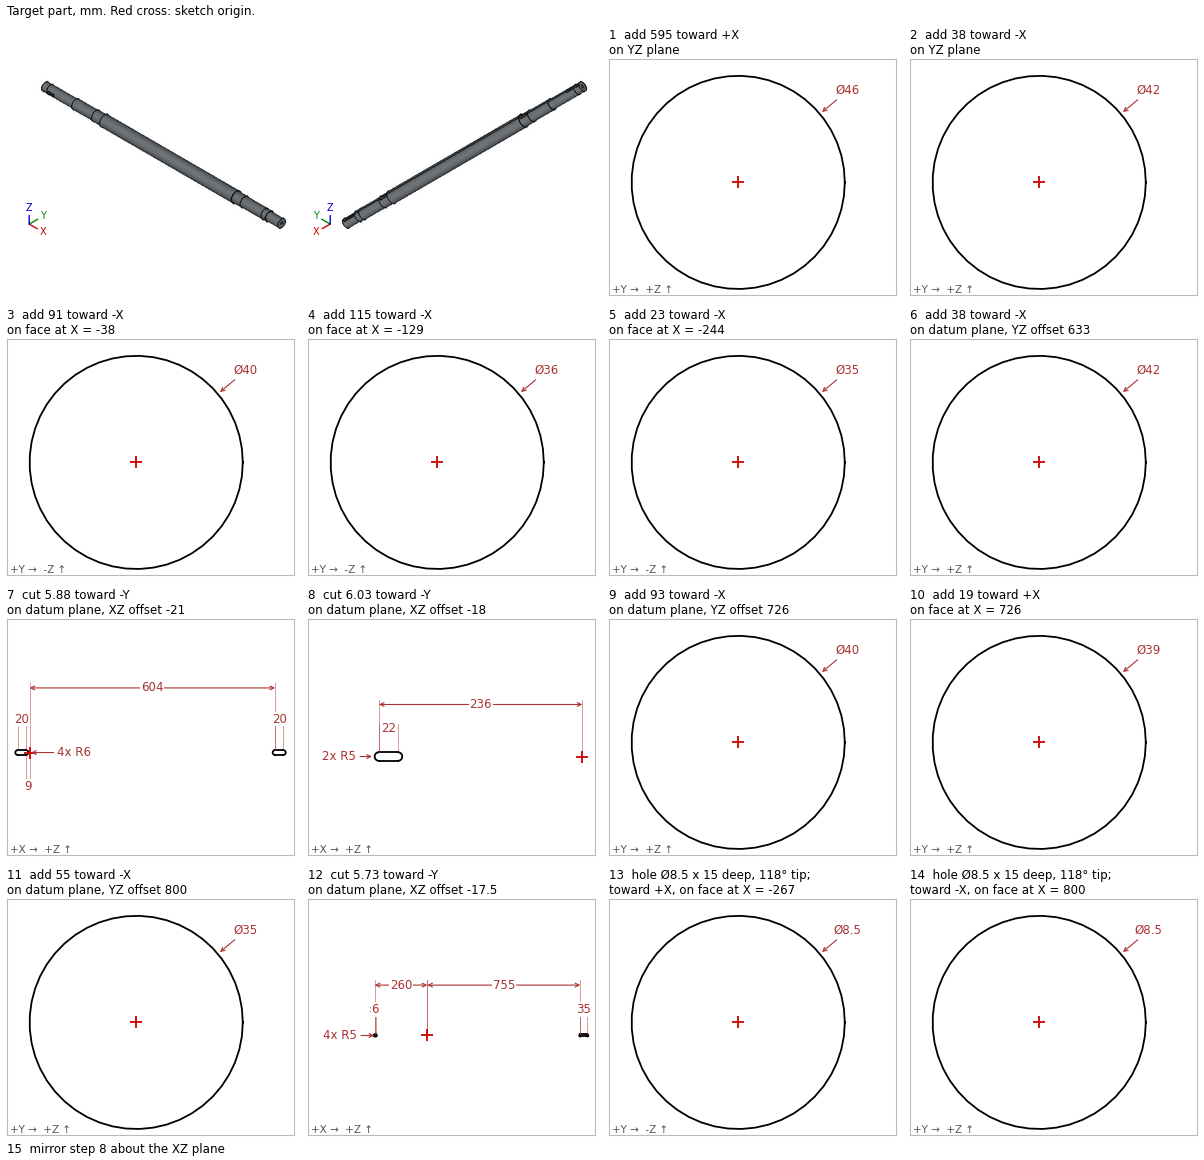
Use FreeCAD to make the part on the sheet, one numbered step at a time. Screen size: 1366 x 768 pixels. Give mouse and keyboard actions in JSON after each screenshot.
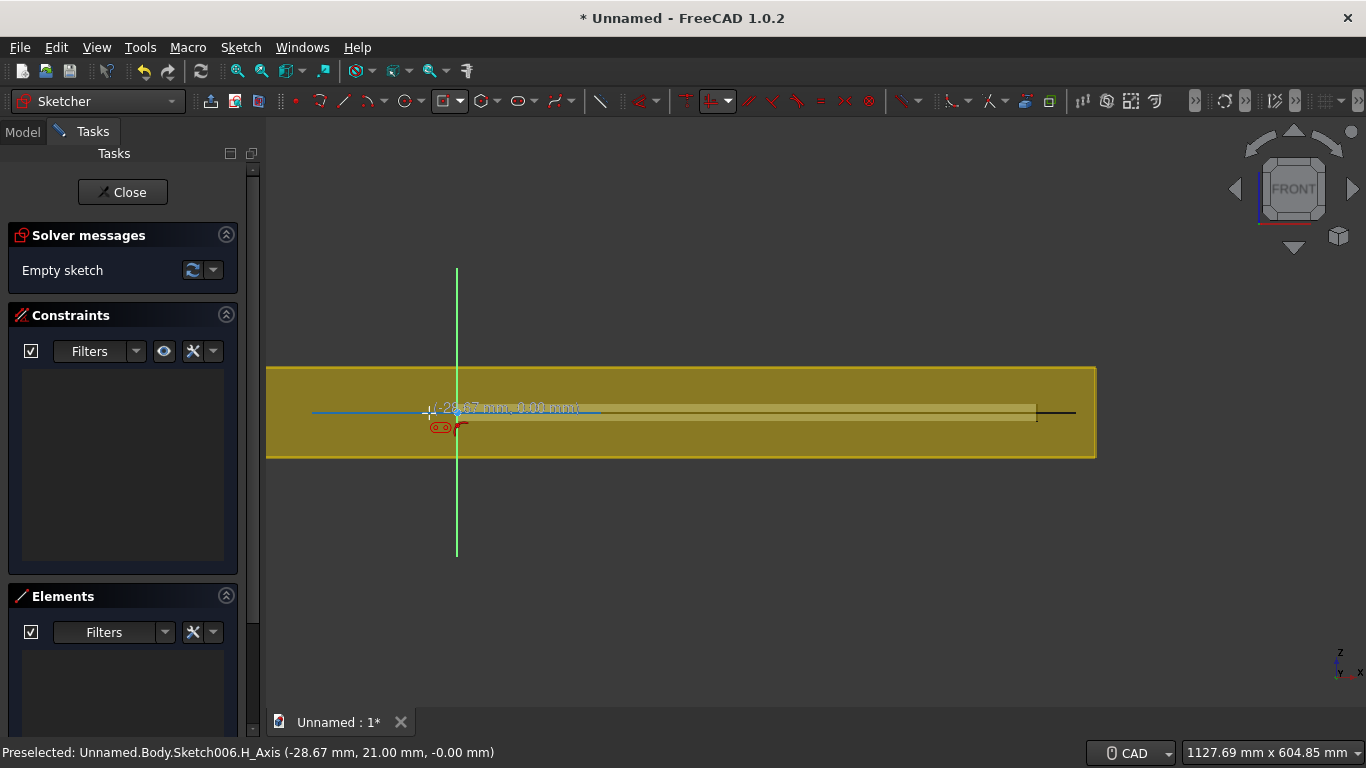
{"action": "left_click", "coordinate": [429, 413]}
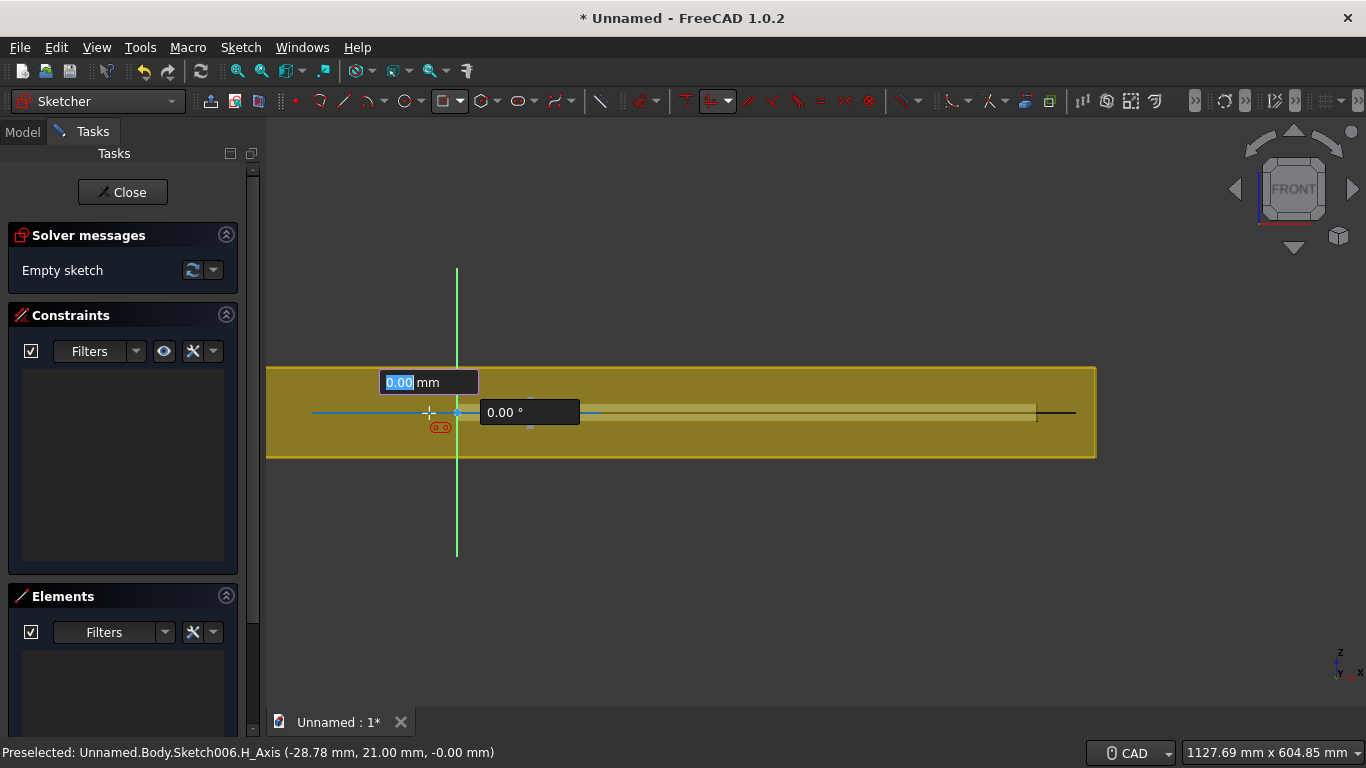
{"action": "scroll", "coordinate": [448, 413], "scroll_direction": "up", "scroll_amount": 3}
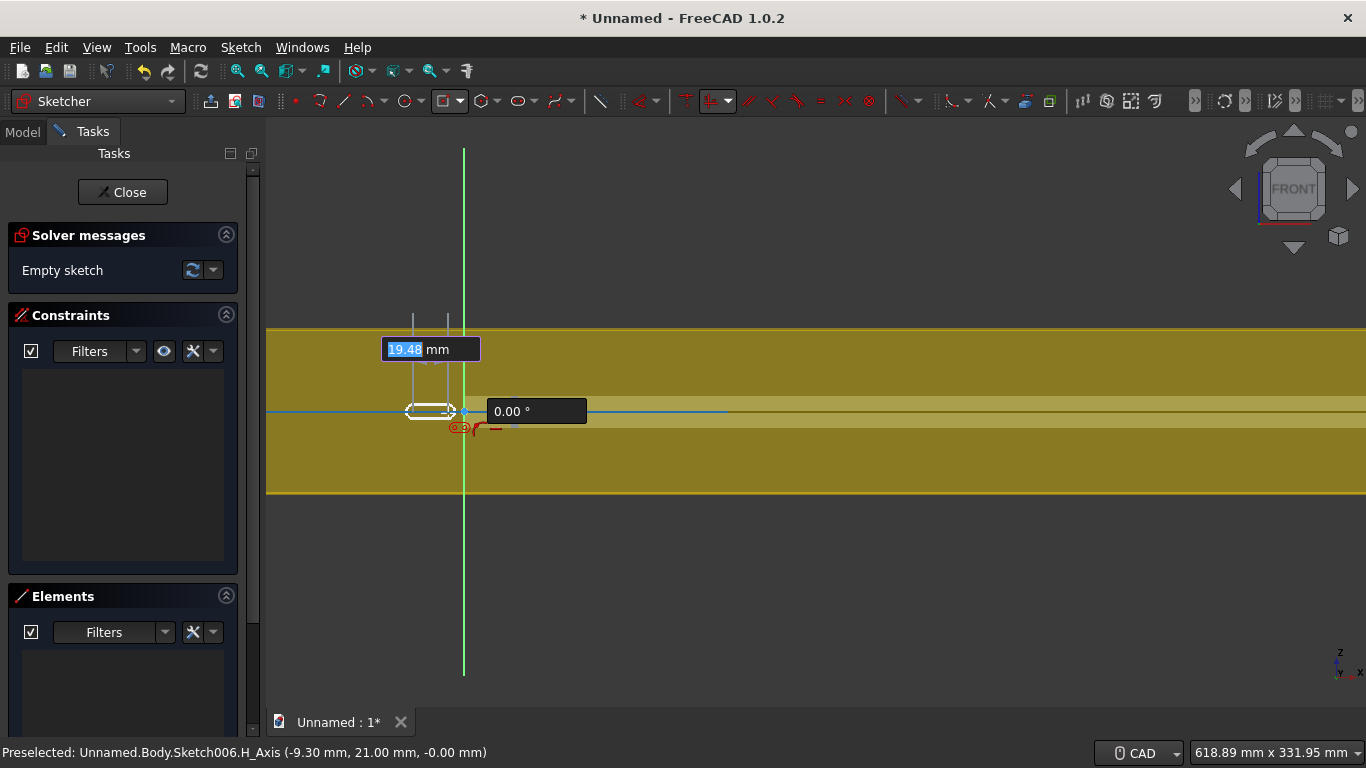
{"action": "left_click", "coordinate": [448, 403]}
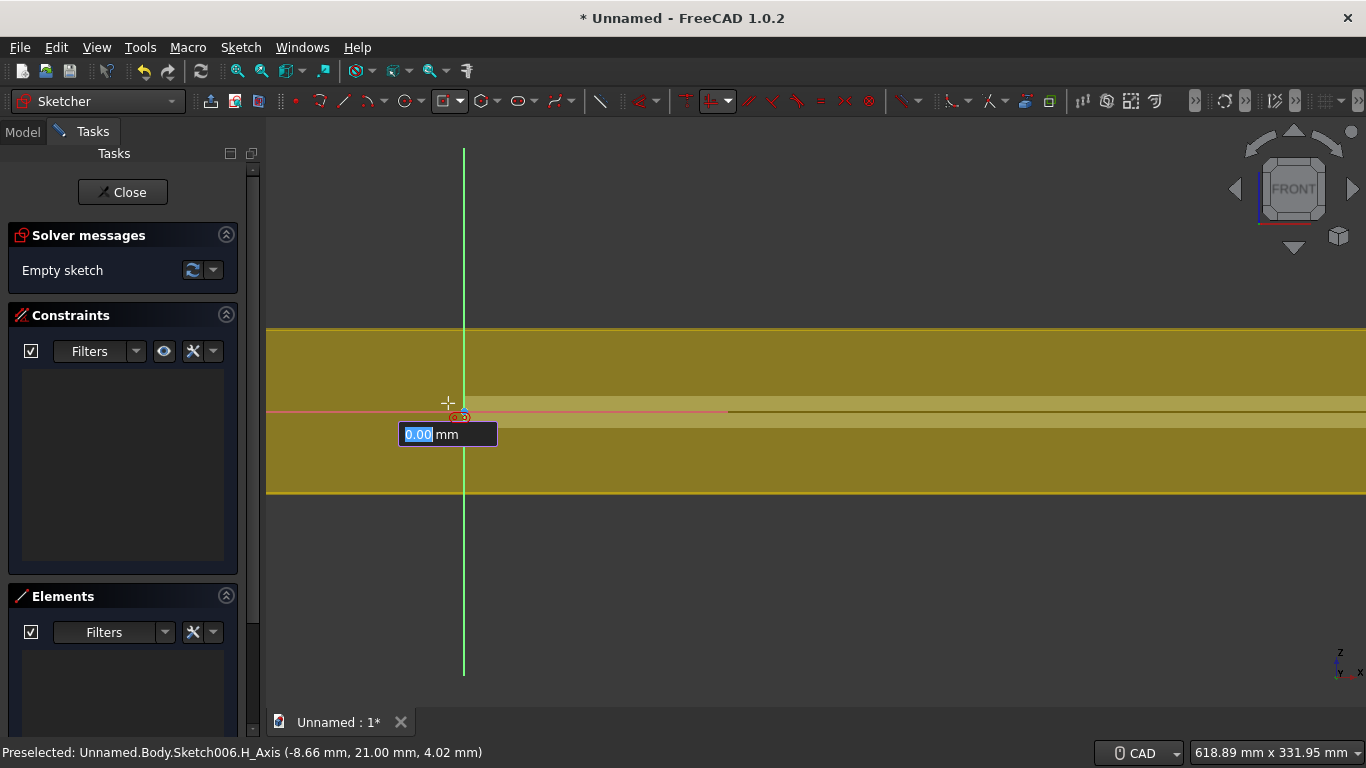
{"action": "scroll", "coordinate": [431, 401], "scroll_direction": "up", "scroll_amount": 2}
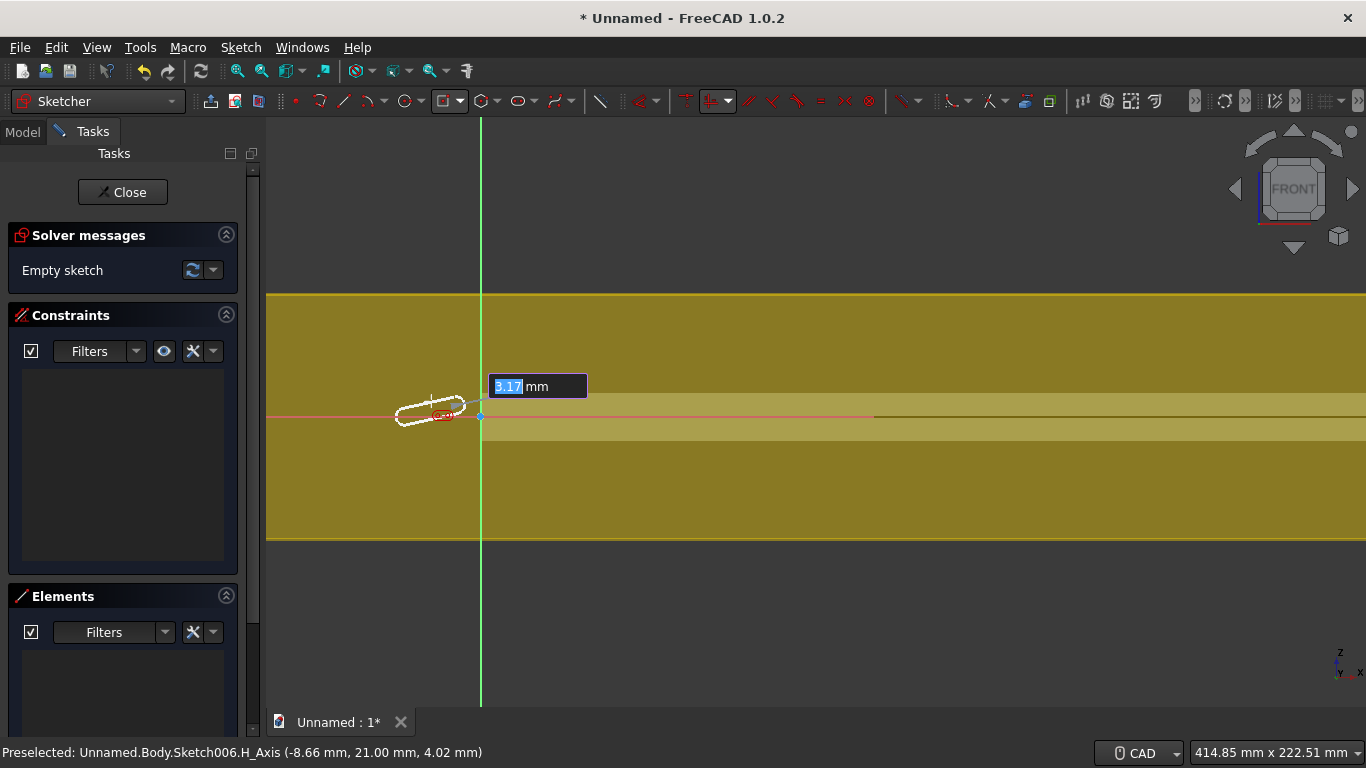
{"action": "left_click", "coordinate": [430, 401]}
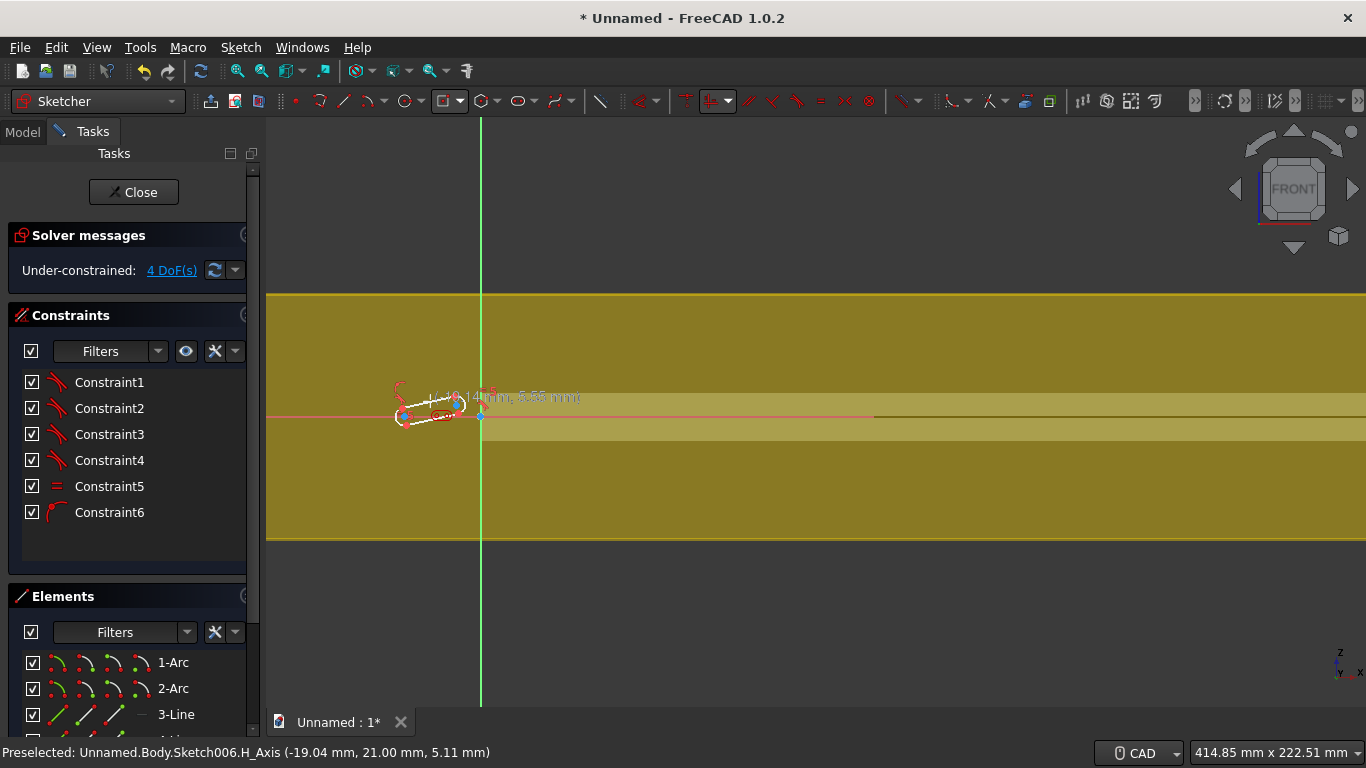
{"action": "scroll", "coordinate": [444, 409], "scroll_direction": "down", "scroll_amount": 5}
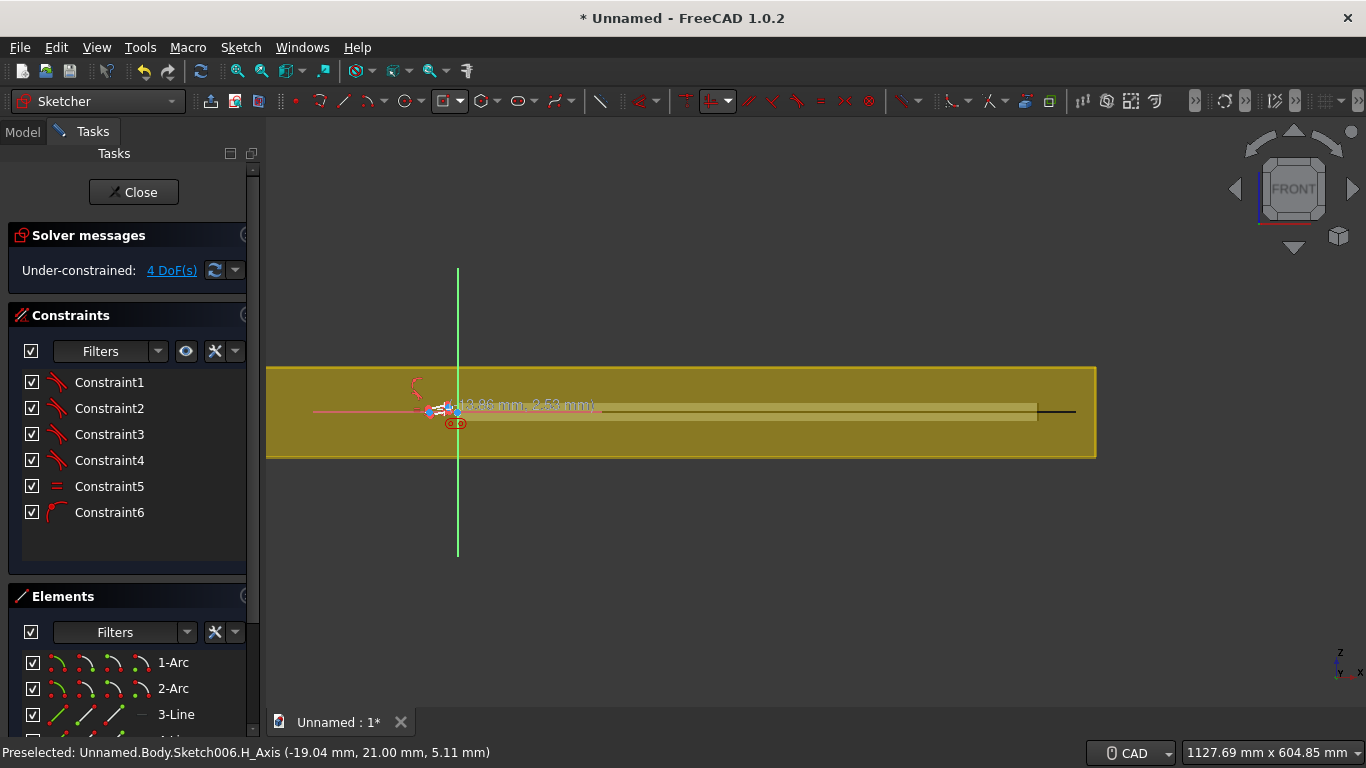
{"action": "scroll", "coordinate": [1047, 412], "scroll_direction": "up", "scroll_amount": 7}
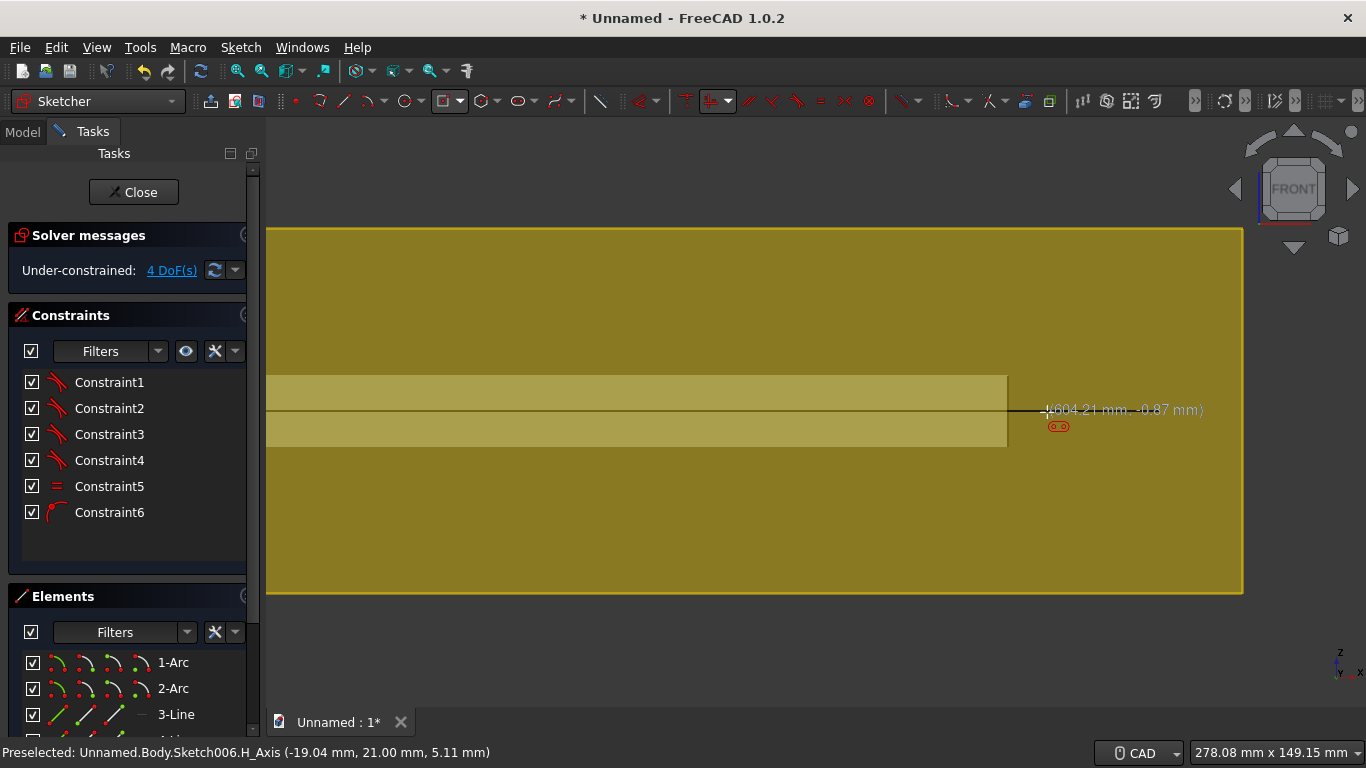
{"action": "scroll", "coordinate": [1047, 412], "scroll_direction": "down", "scroll_amount": 7}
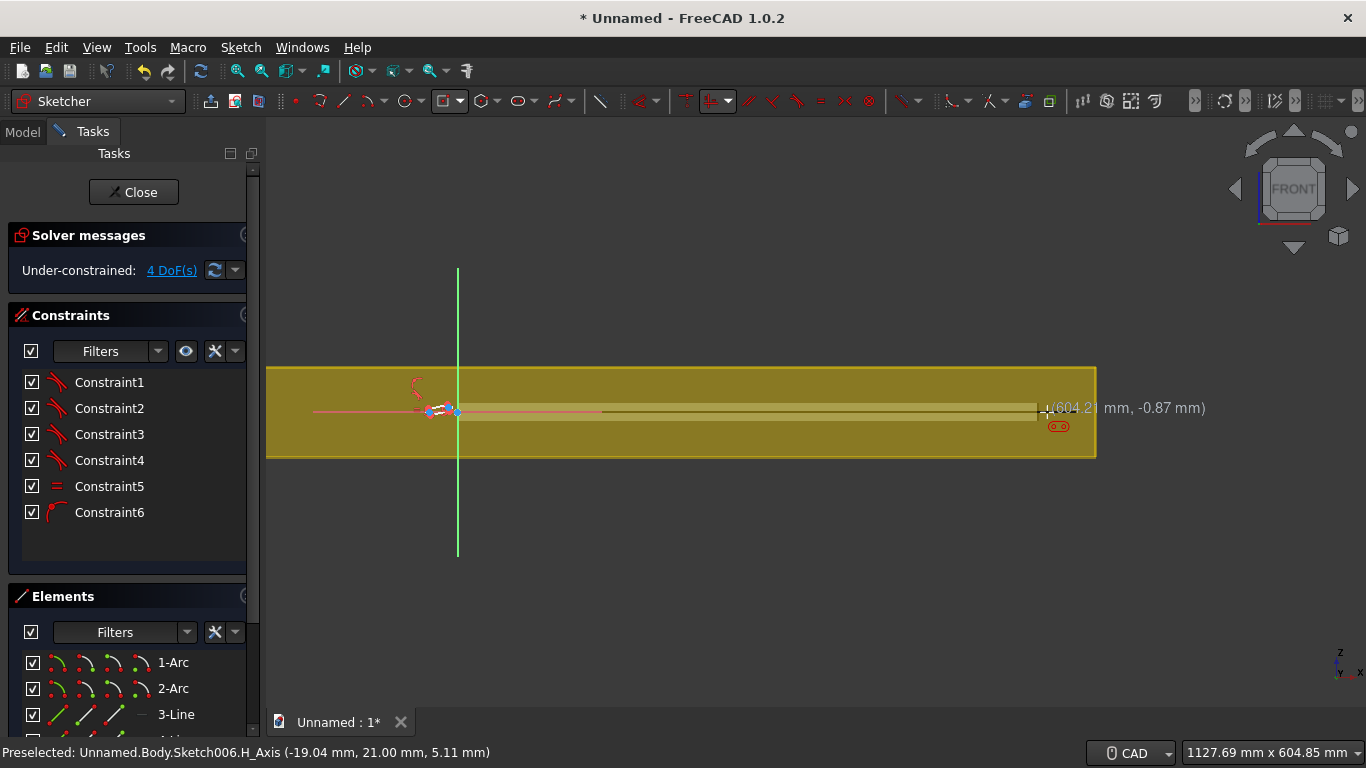
{"action": "left_click", "coordinate": [1047, 412]}